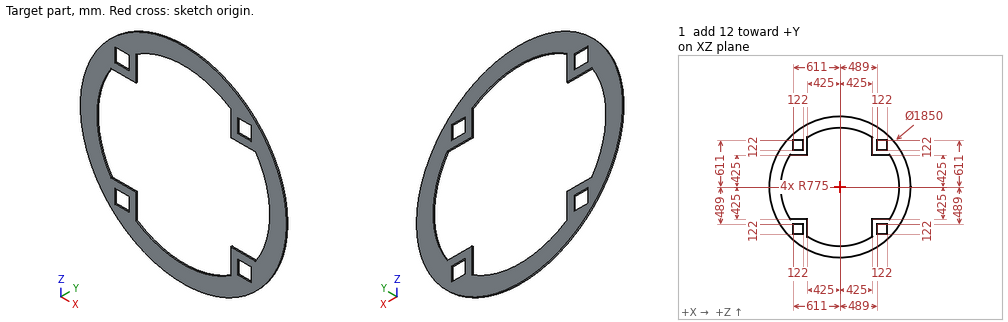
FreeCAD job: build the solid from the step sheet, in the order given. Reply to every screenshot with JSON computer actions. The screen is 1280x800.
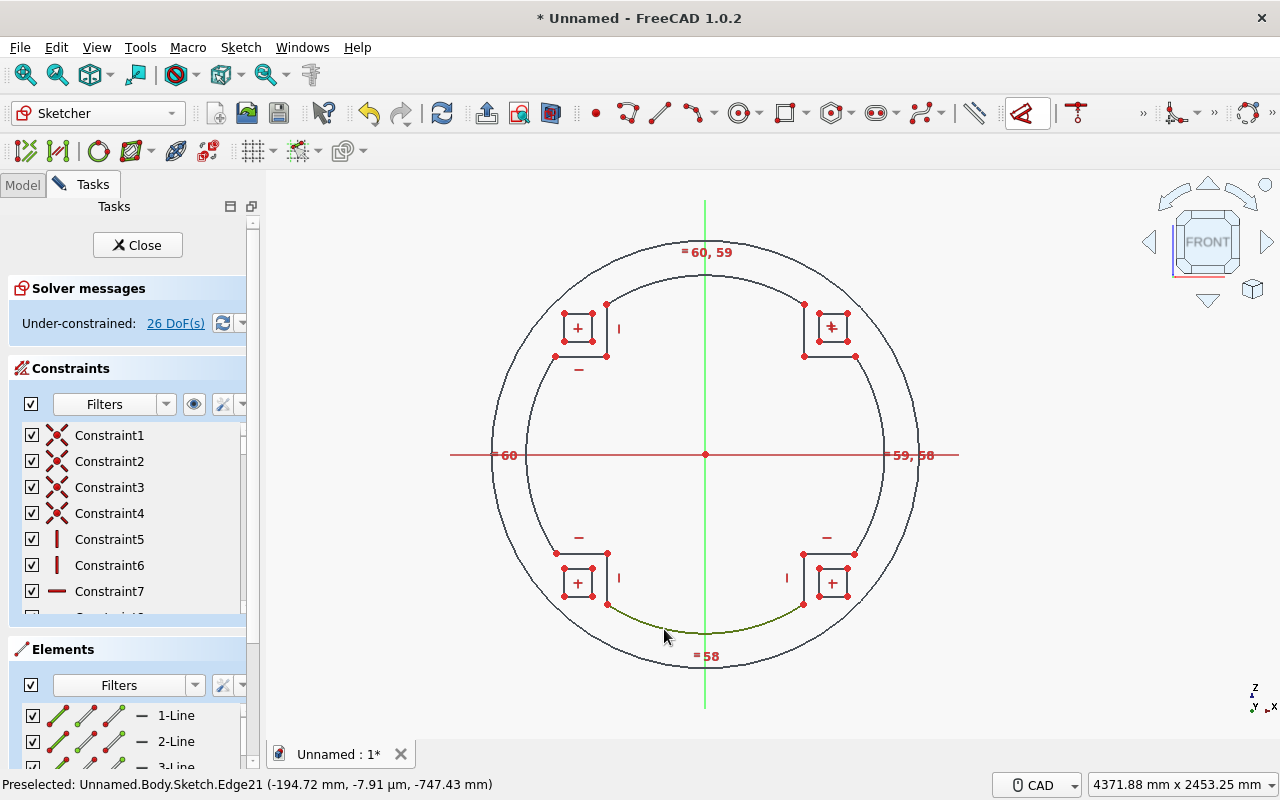
{"action": "key", "text": "k r"}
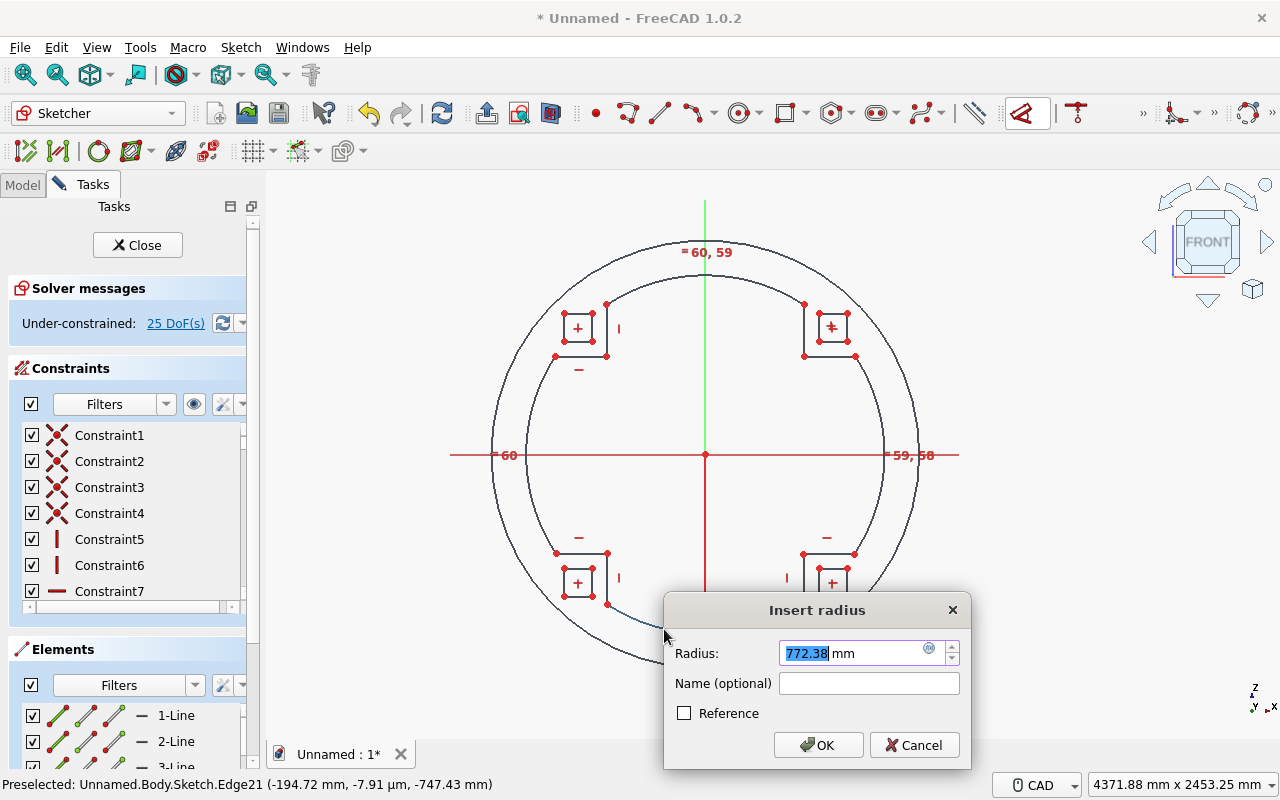
{"action": "type", "text": "775"}
{"action": "key", "text": "Return"}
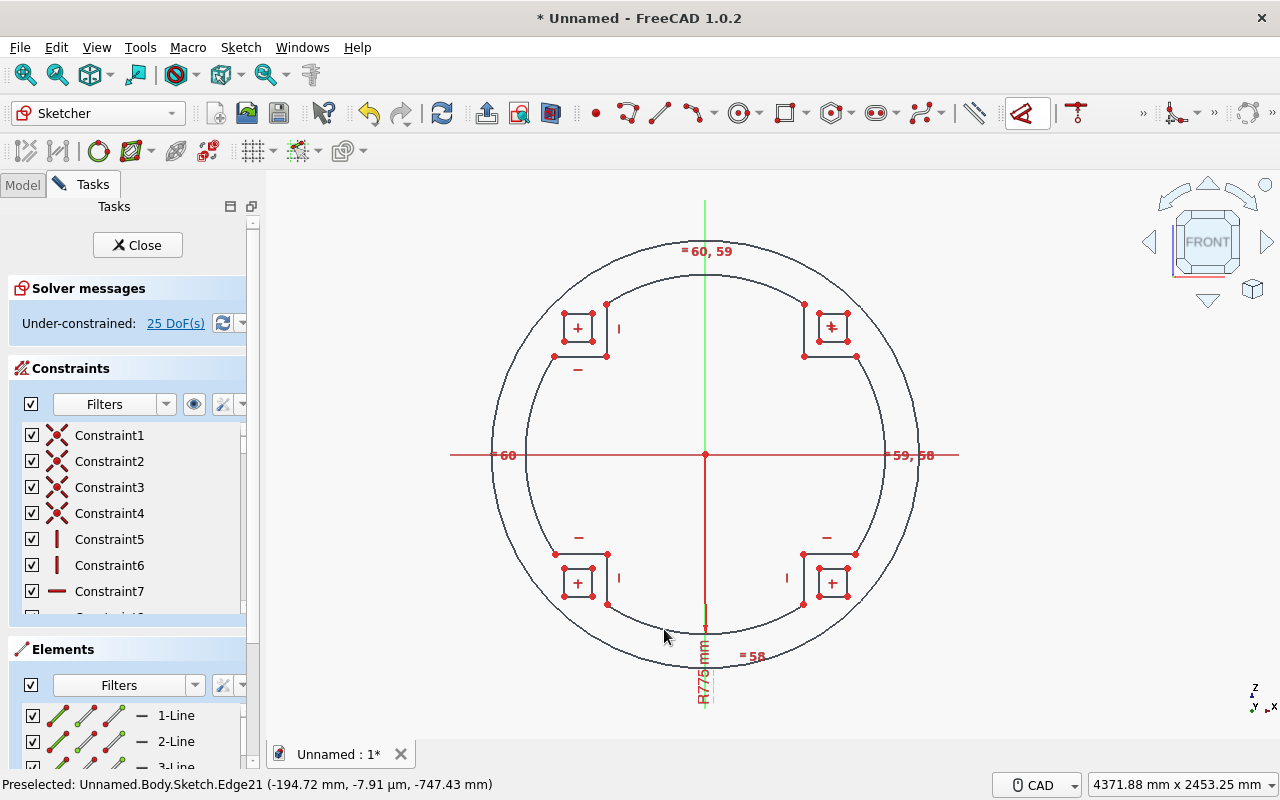
{"action": "left_click", "coordinate": [856, 303]}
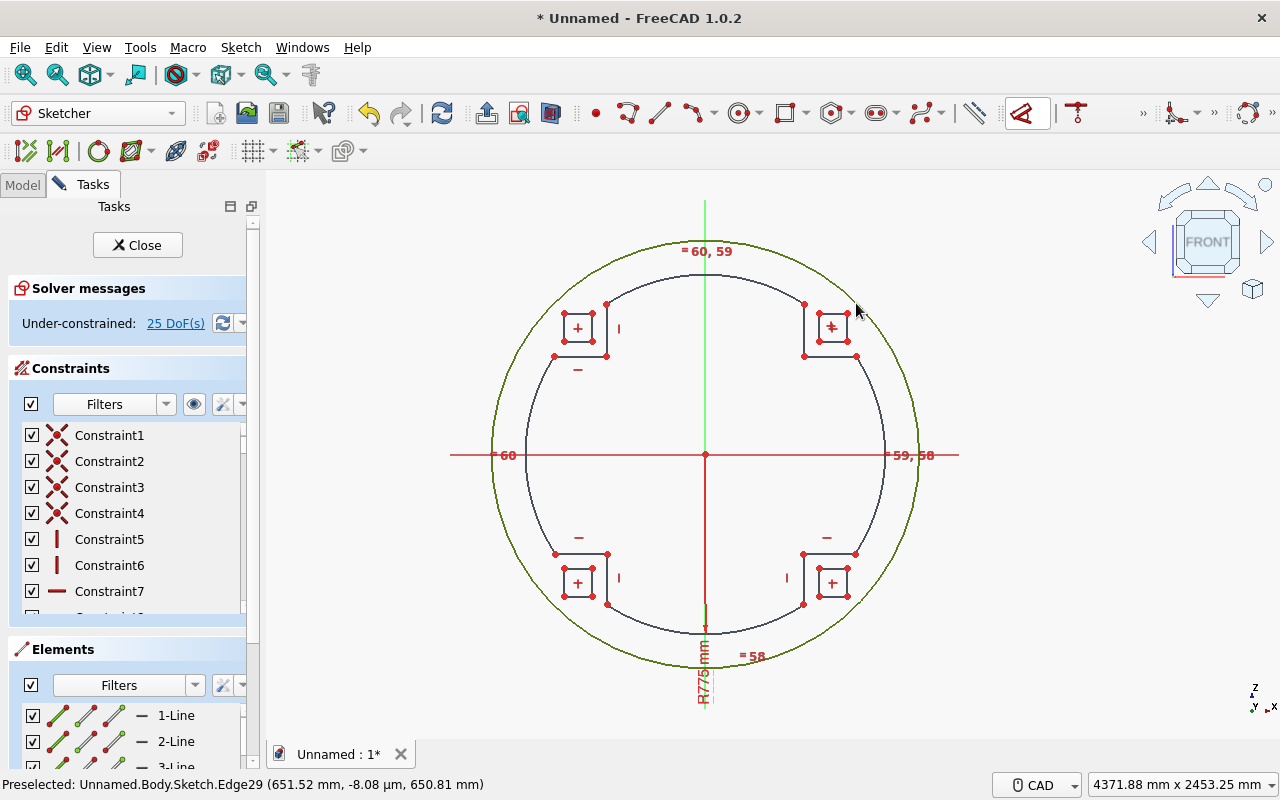
{"action": "key", "text": "k o"}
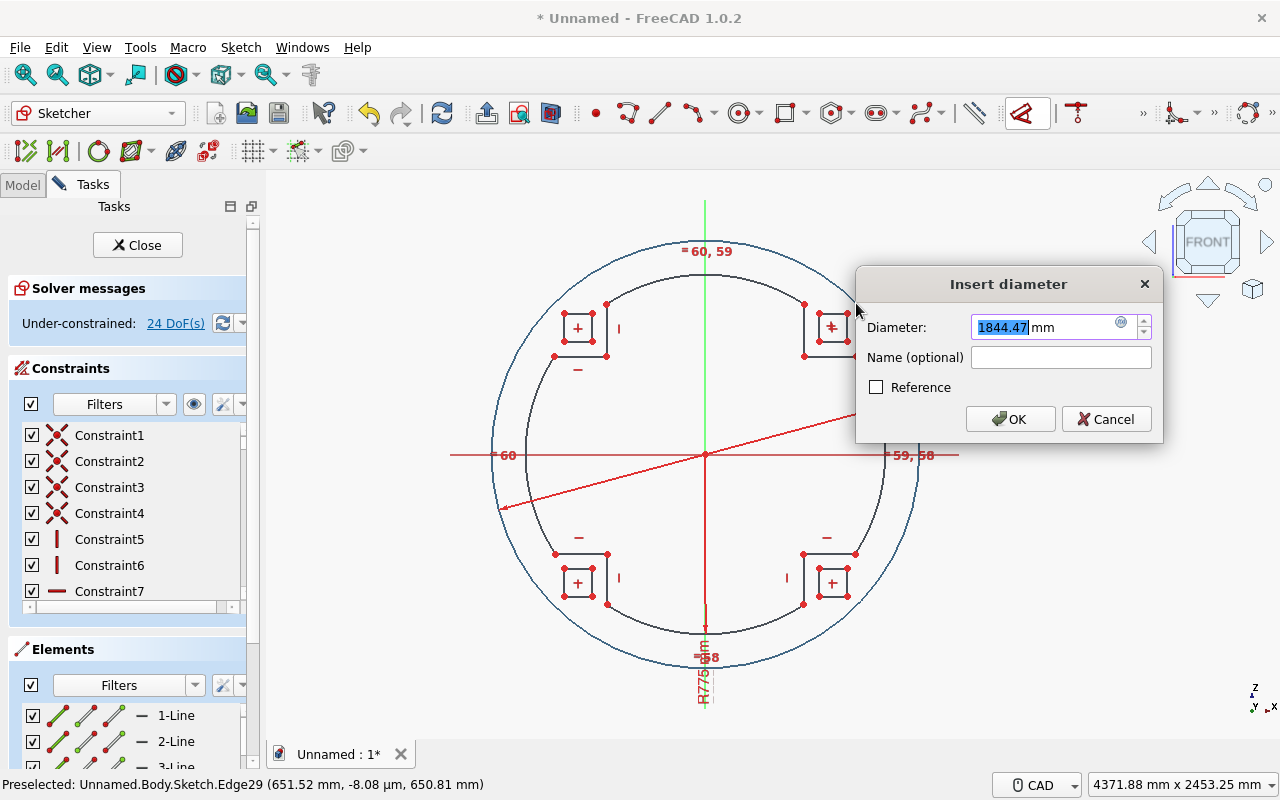
{"action": "type", "text": "1850"}
{"action": "key", "text": "Return"}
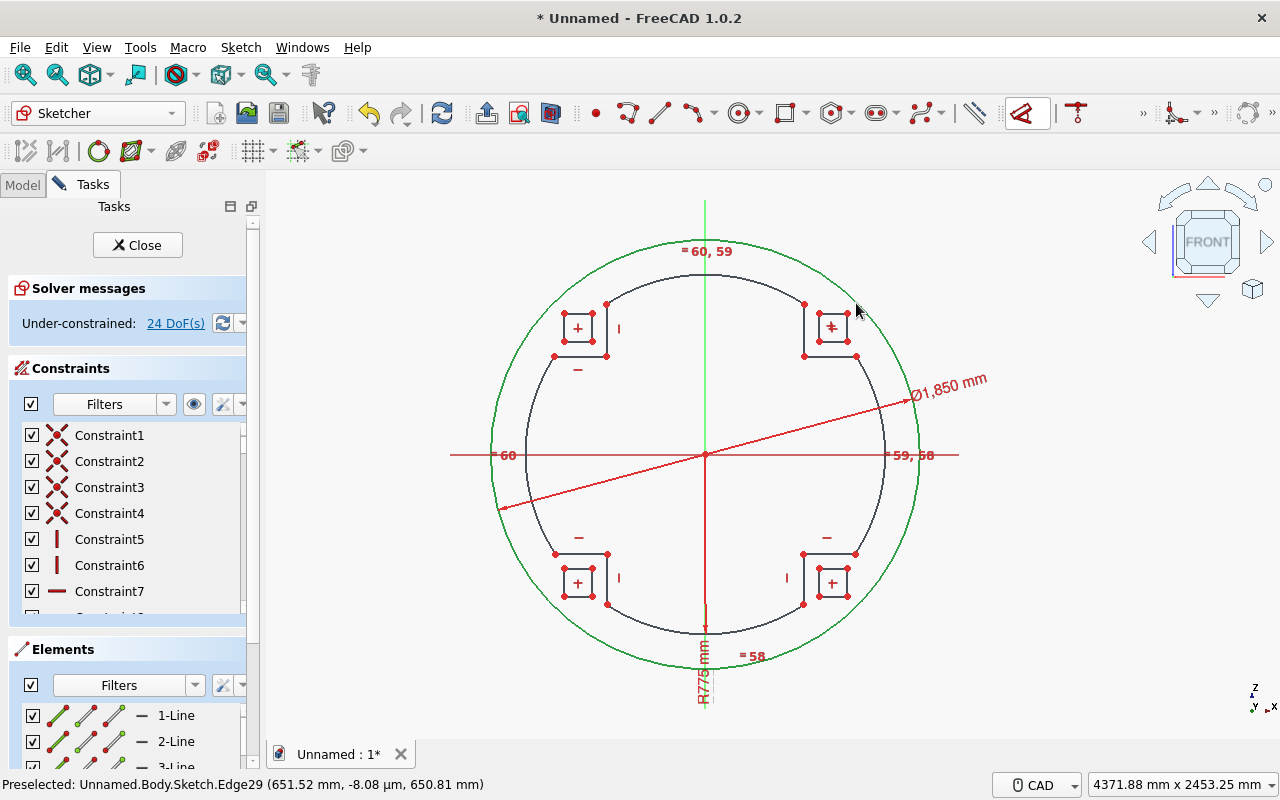
{"action": "scroll", "coordinate": [564, 580], "scroll_direction": "up", "scroll_amount": 2}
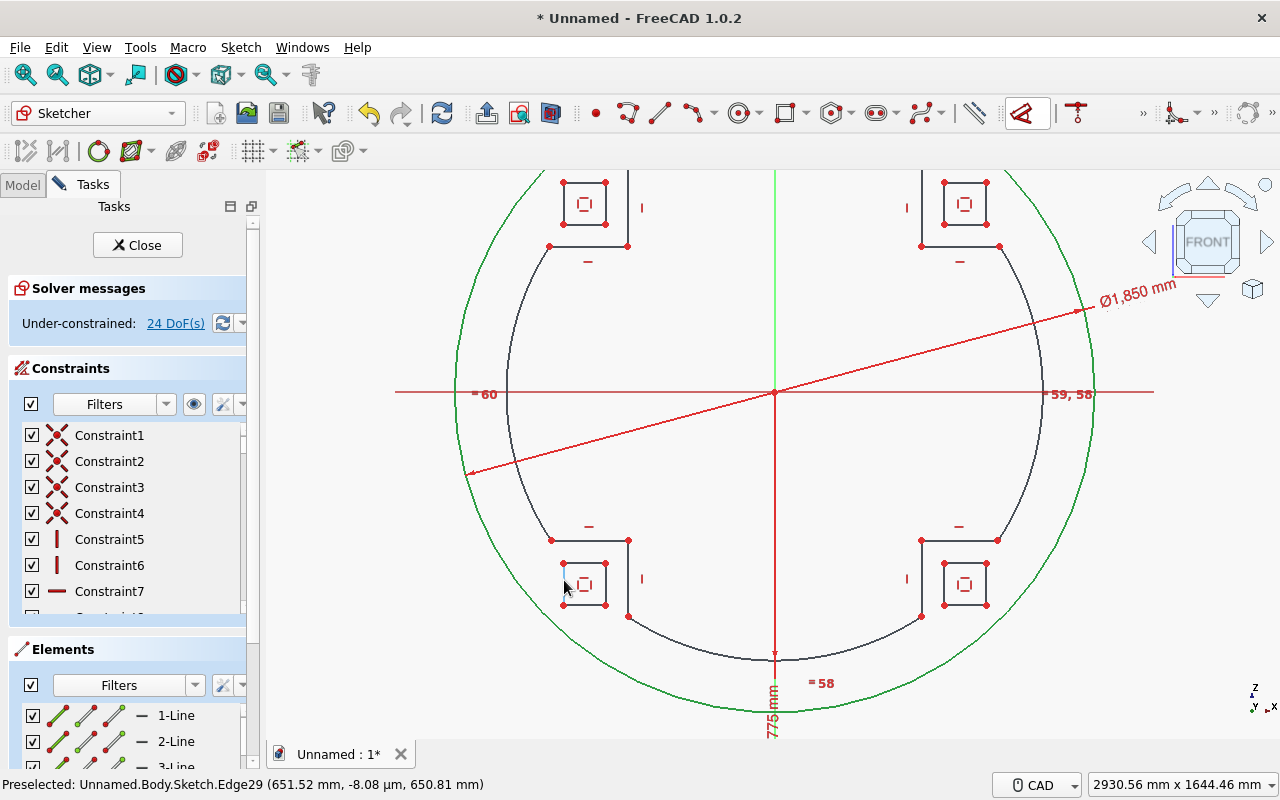
{"action": "left_click", "coordinate": [564, 580]}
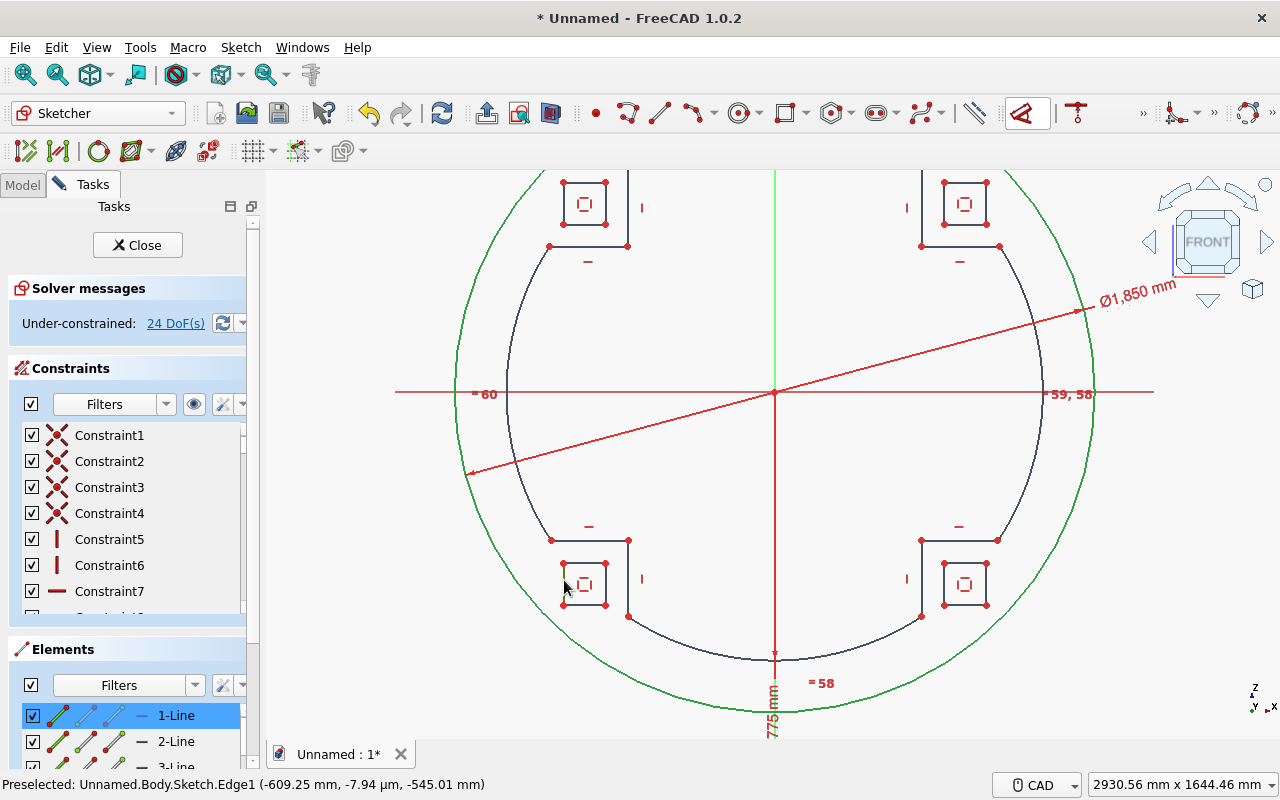
{"action": "key", "text": "i"}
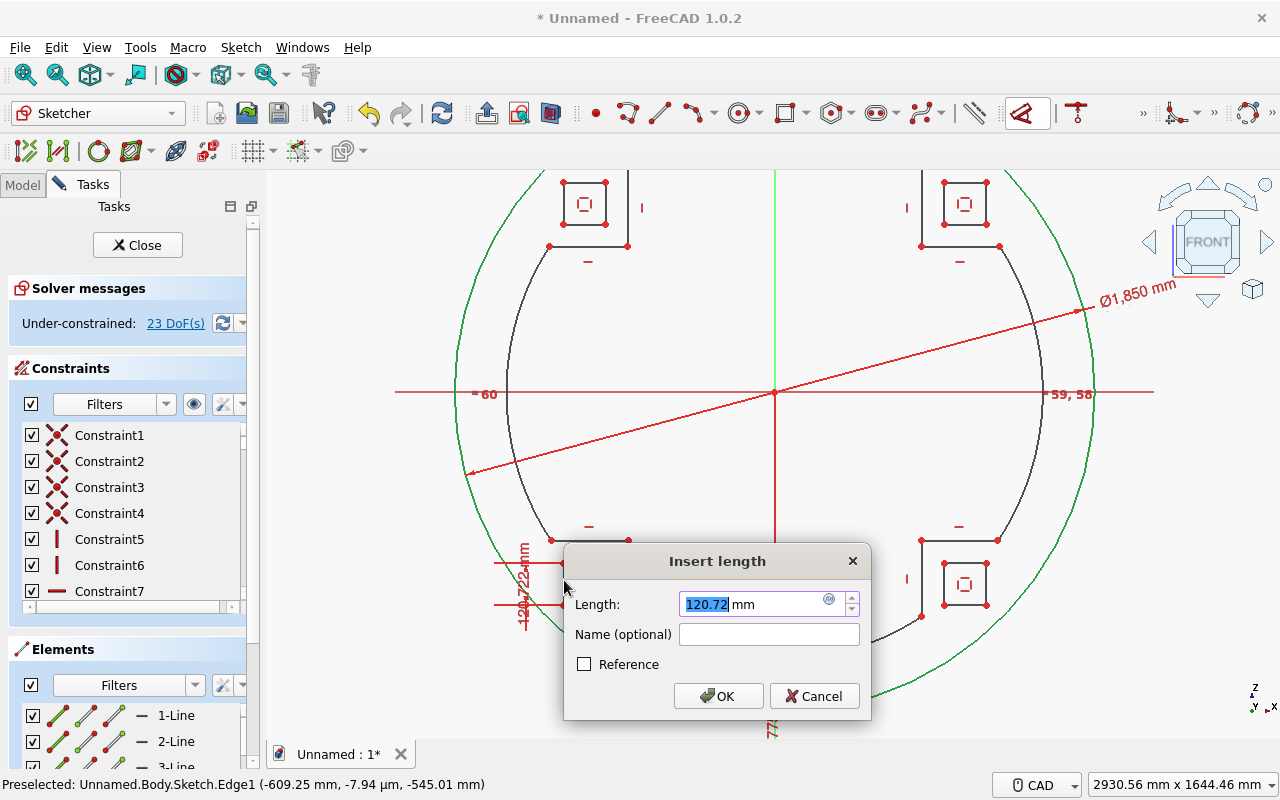
{"action": "type", "text": "122"}
{"action": "key", "text": "Return"}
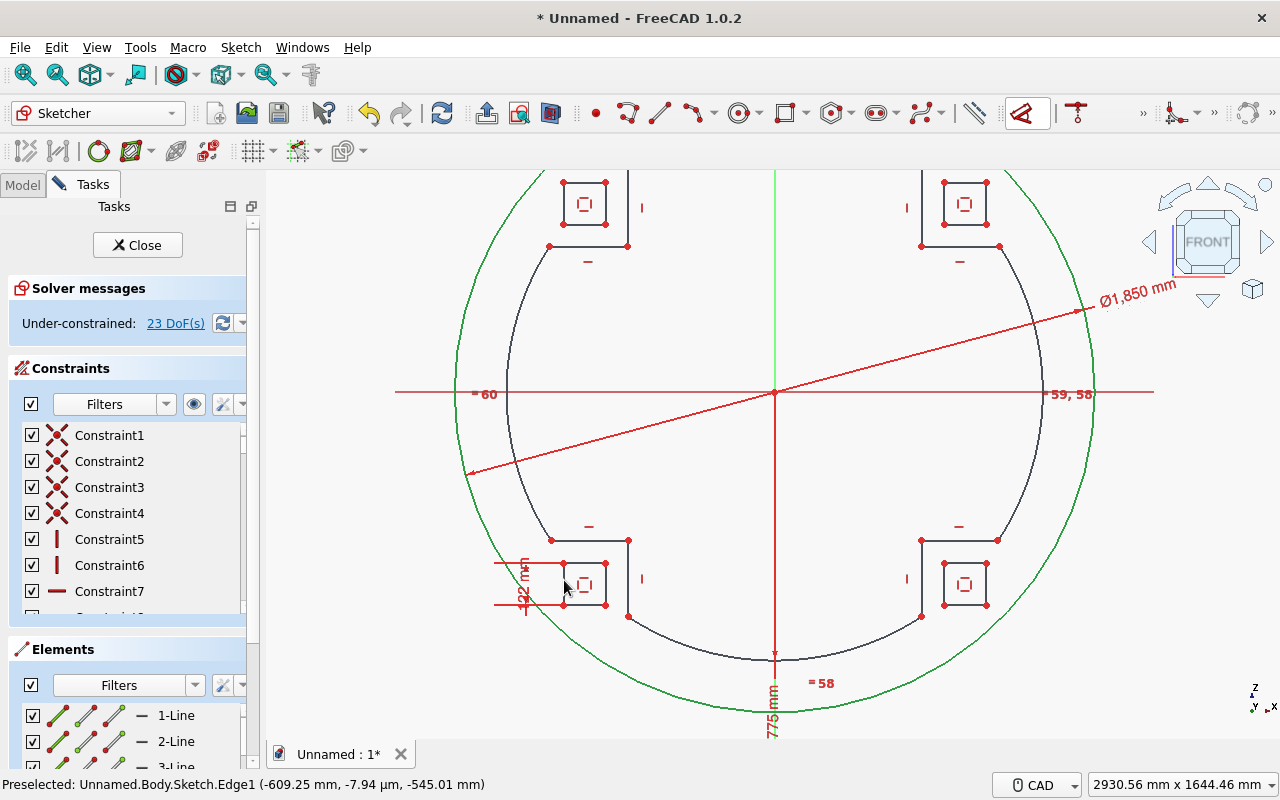
{"action": "left_click", "coordinate": [576, 605]}